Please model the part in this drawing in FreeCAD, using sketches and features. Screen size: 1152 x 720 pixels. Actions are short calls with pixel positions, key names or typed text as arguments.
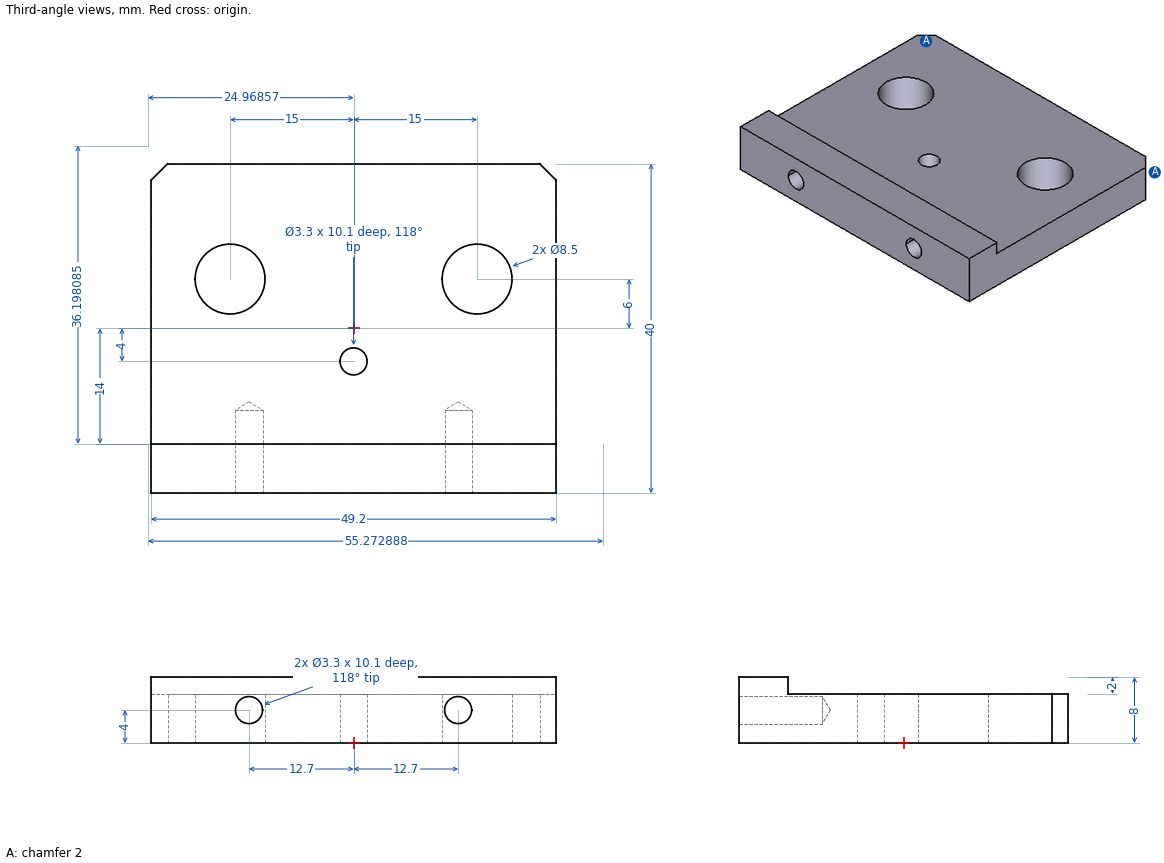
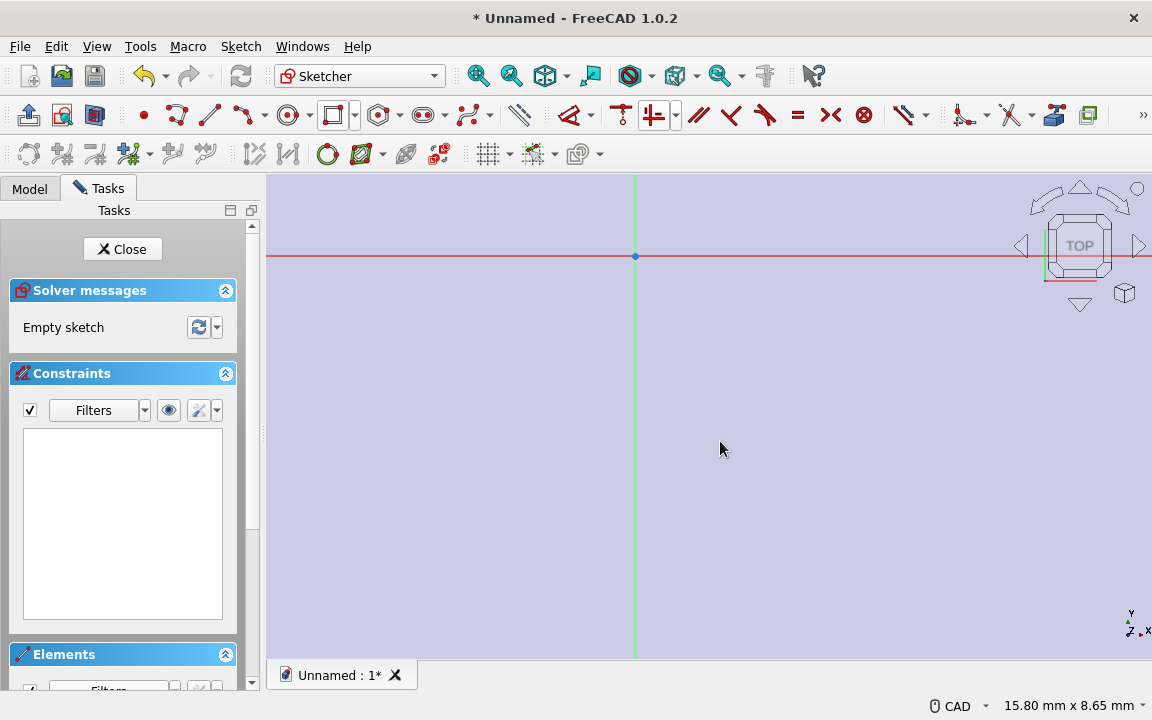
key(g)
key(c)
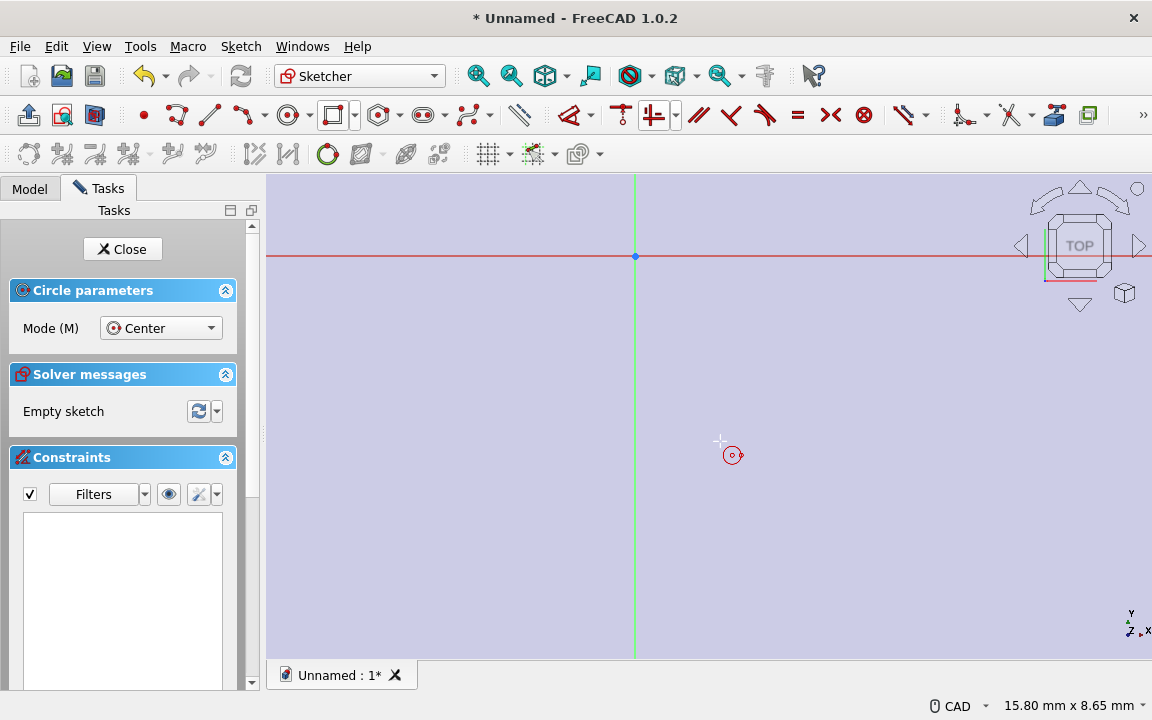
click(635, 481)
click(701, 415)
key(Escape)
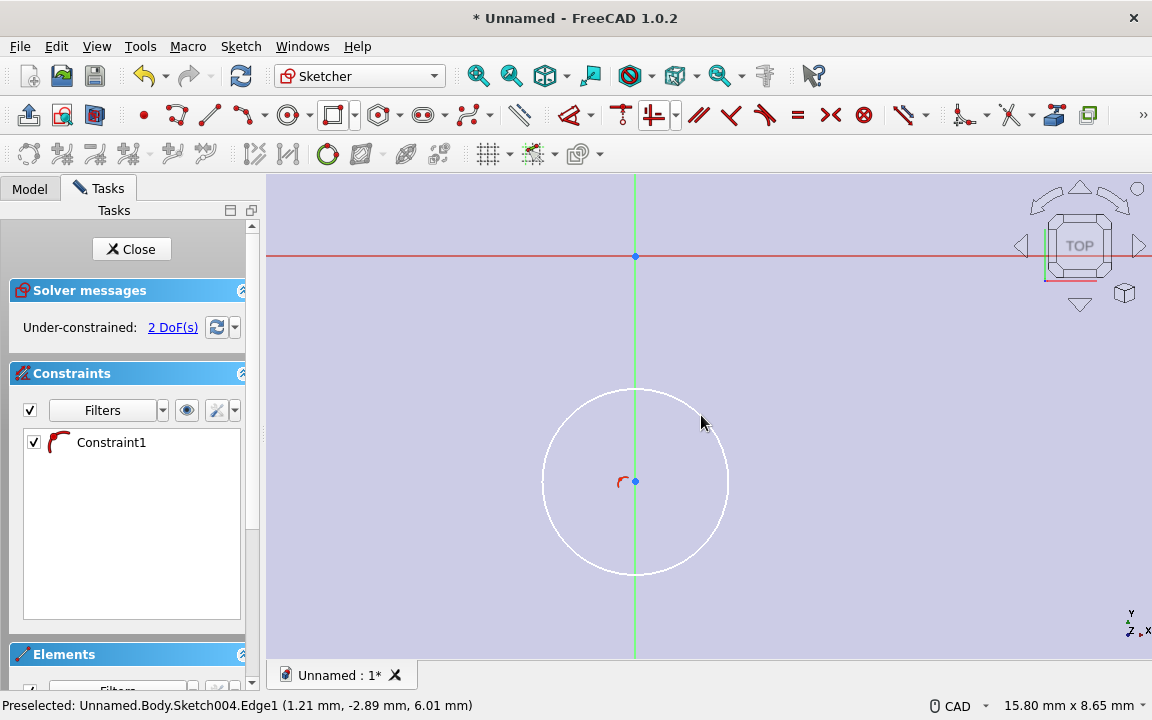
key(d)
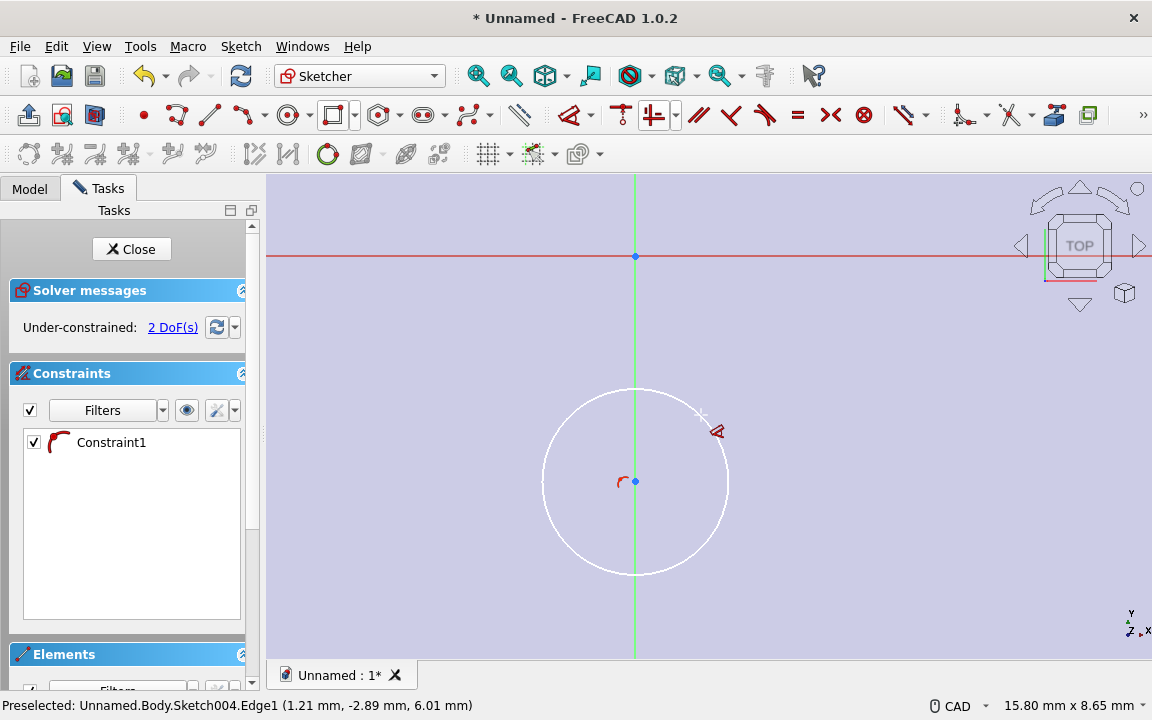
click(701, 416)
click(724, 393)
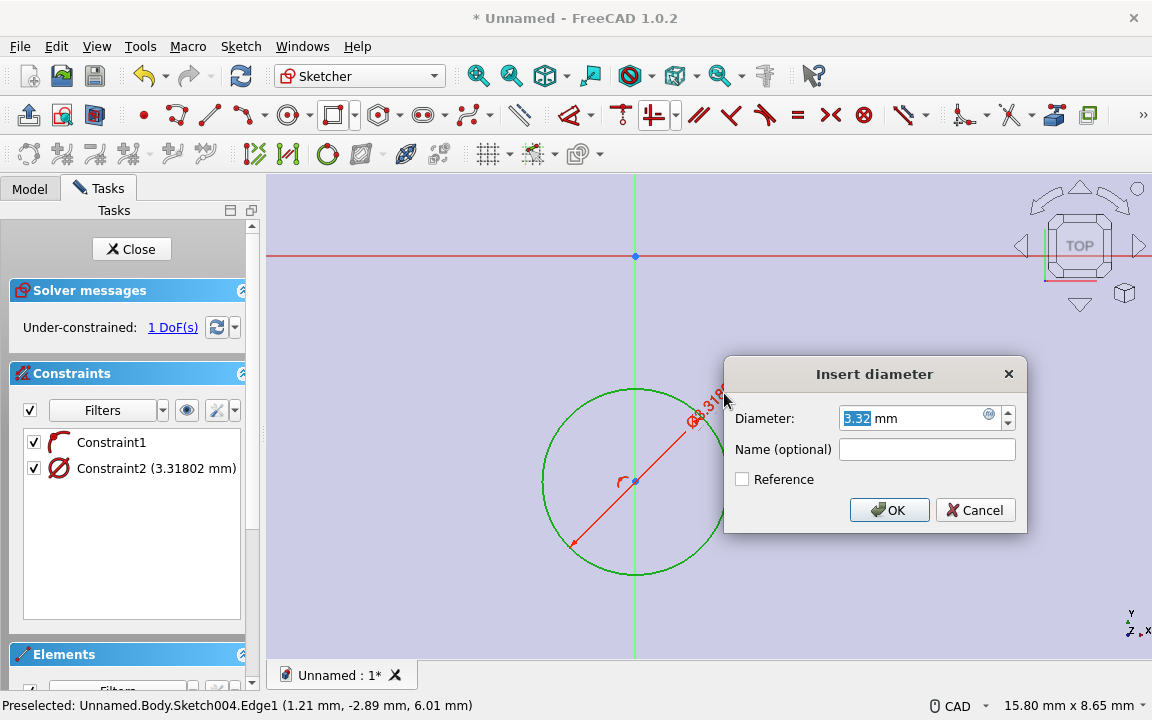
text(3.3)
key(Return)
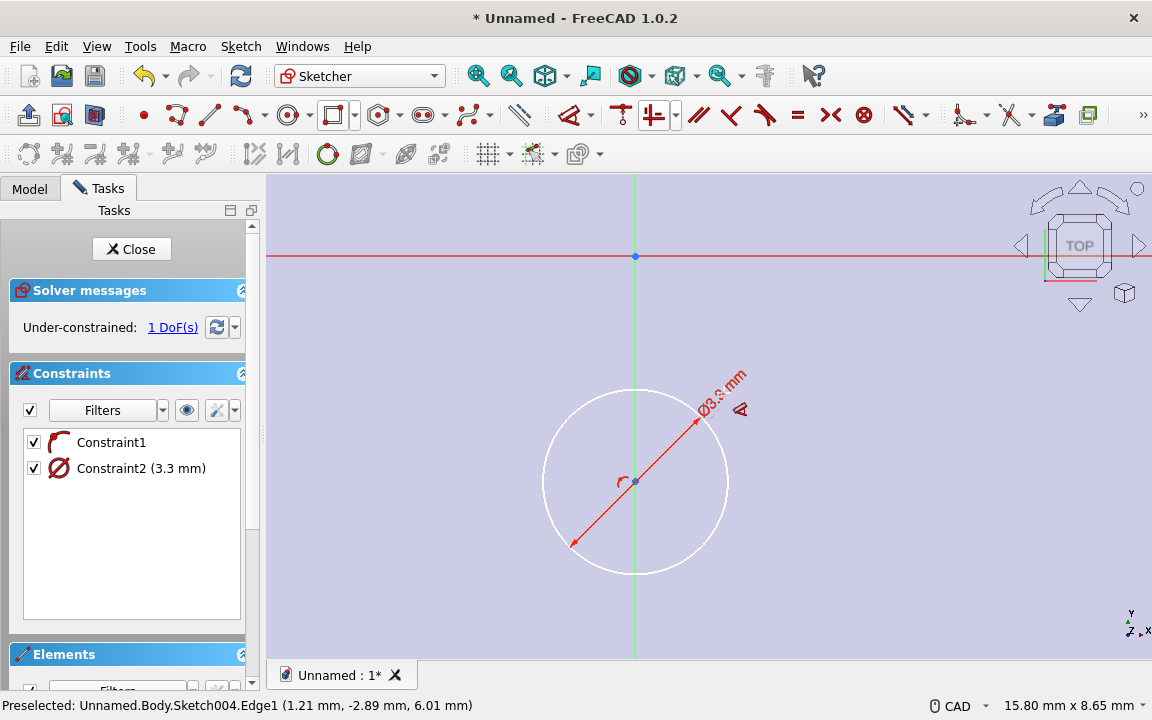
click(635, 482)
click(669, 369)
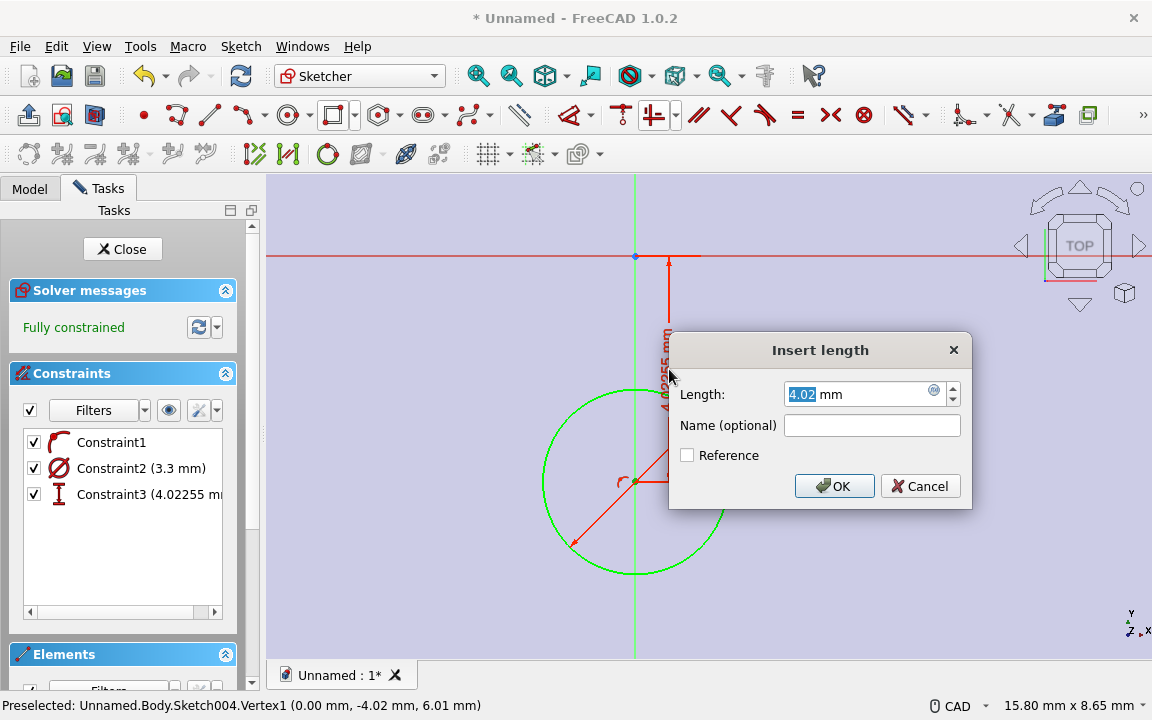
text(4)
key(Return)
key(Escape)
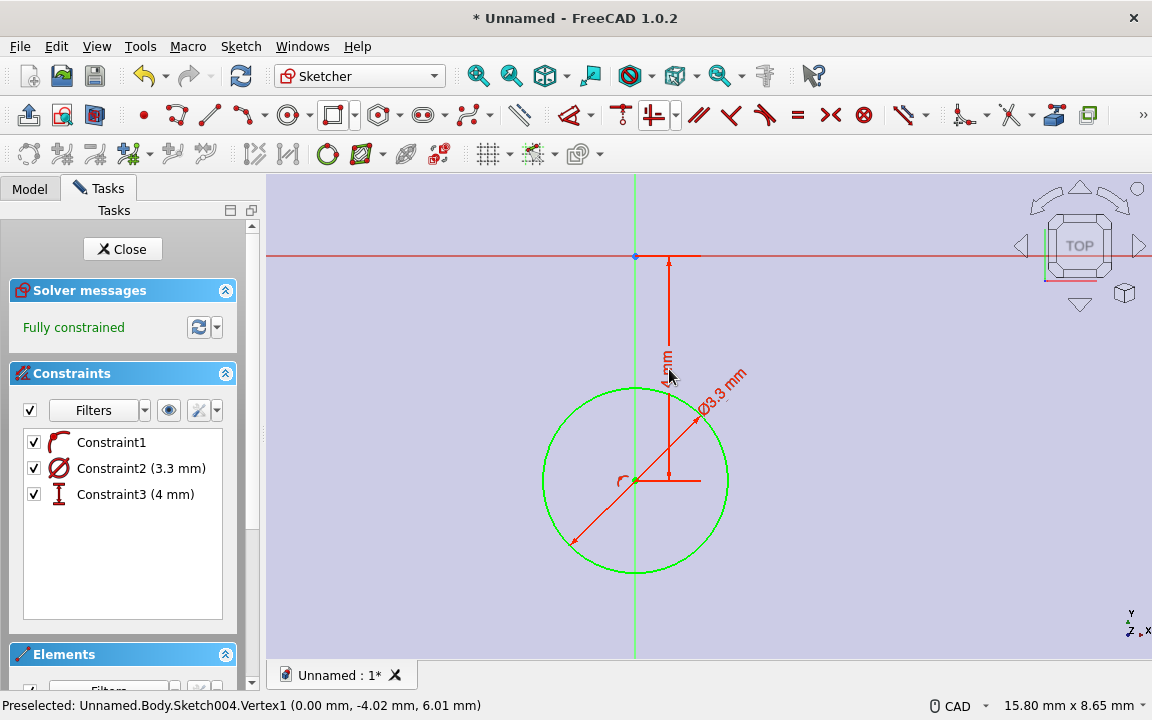
click(123, 249)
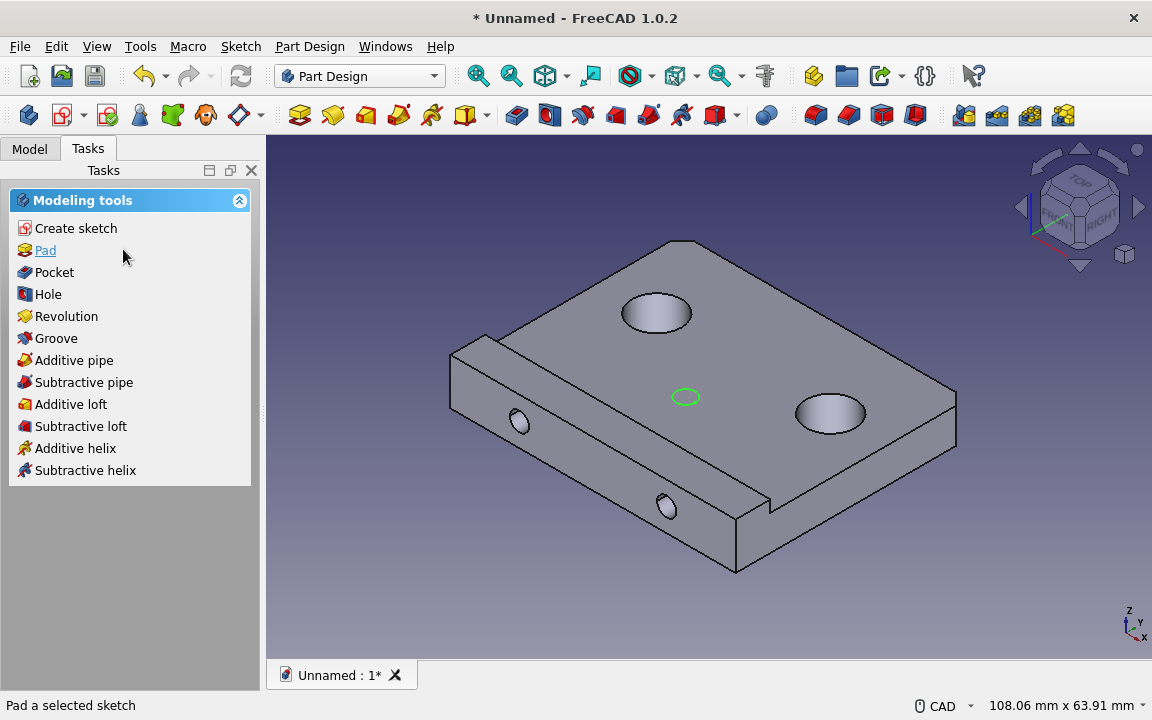
click(550, 116)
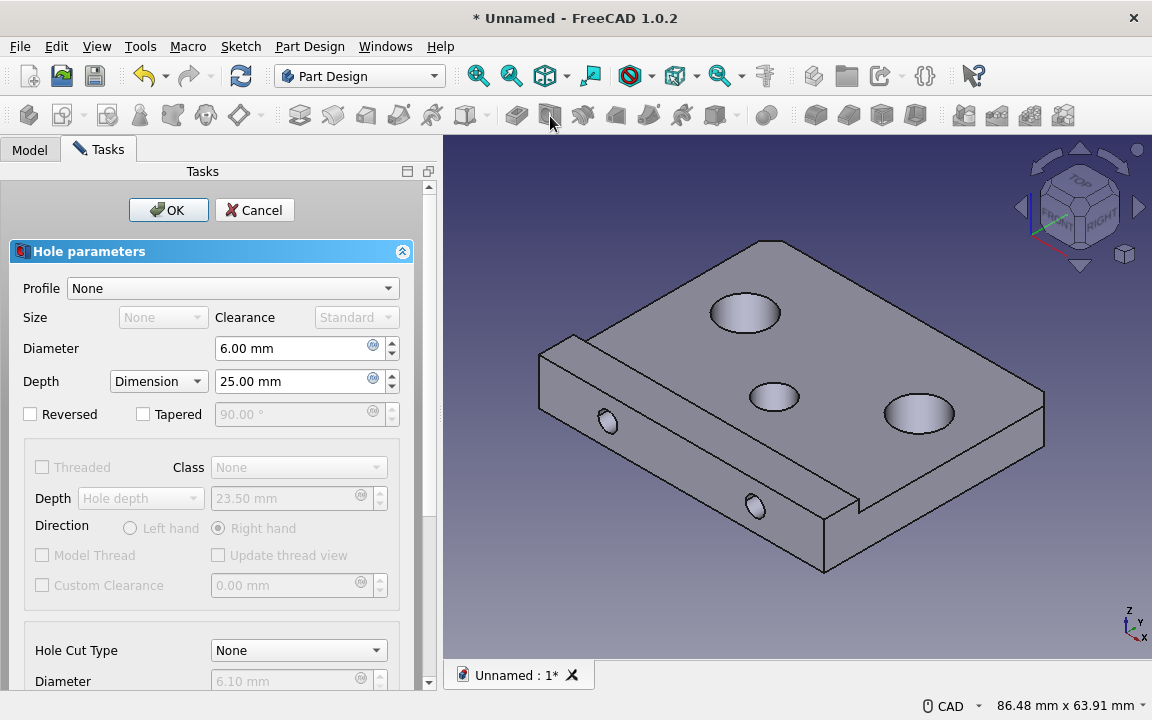
triple_click(300, 348)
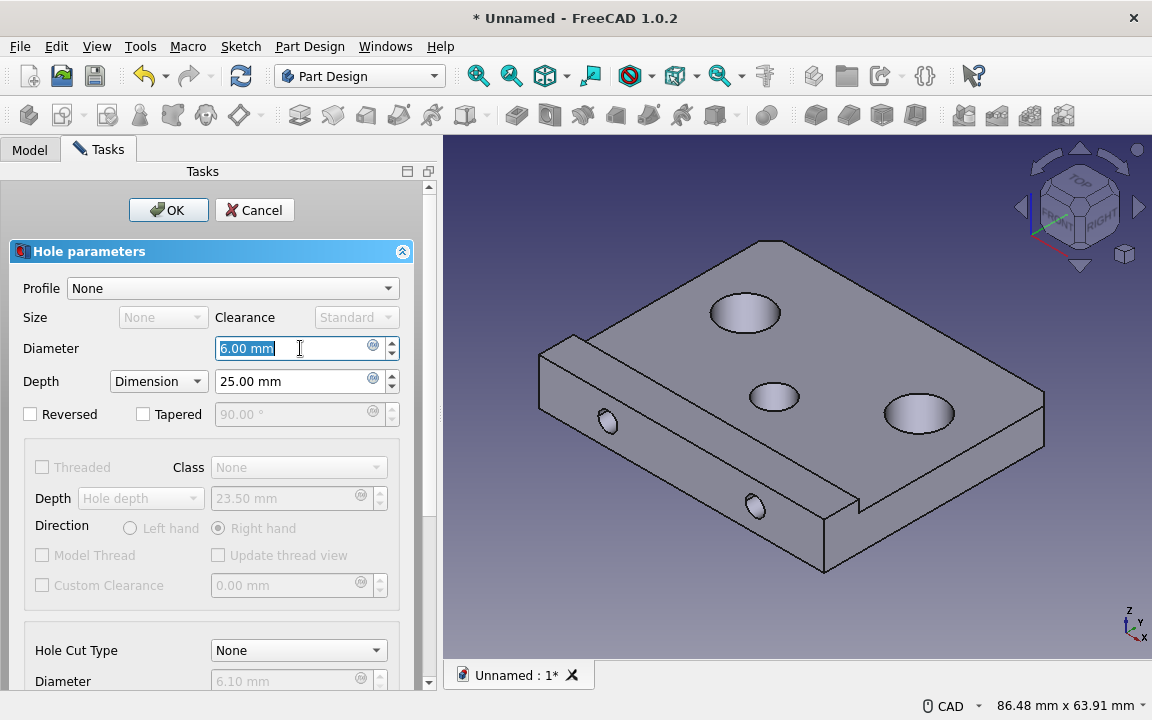
text(3.3)
key(Tab)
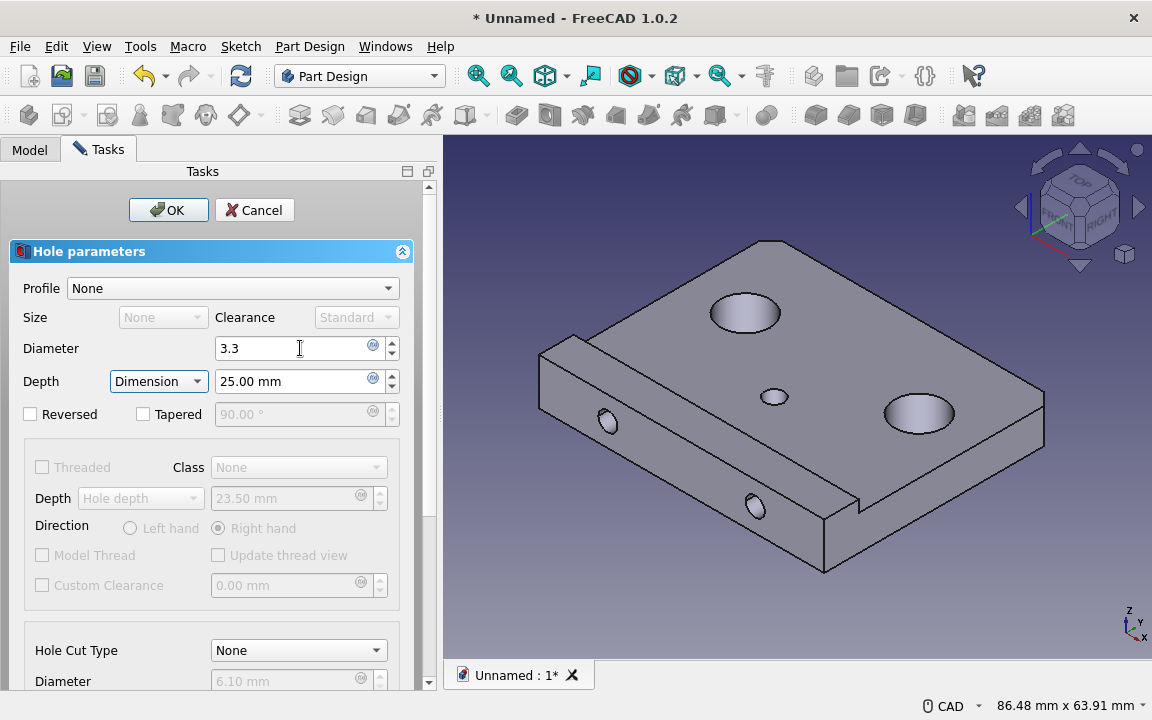
triple_click(300, 382)